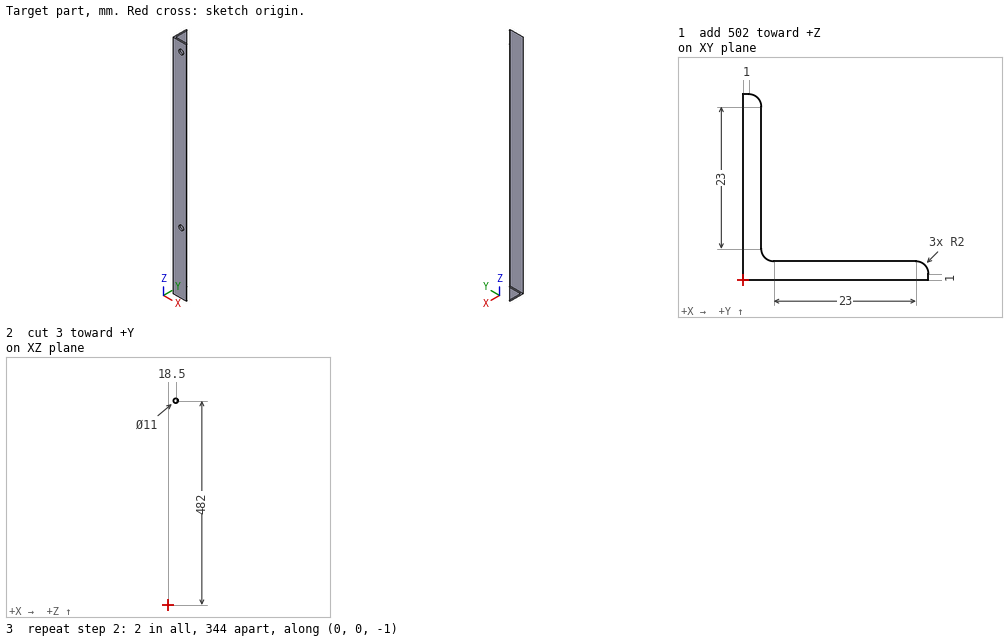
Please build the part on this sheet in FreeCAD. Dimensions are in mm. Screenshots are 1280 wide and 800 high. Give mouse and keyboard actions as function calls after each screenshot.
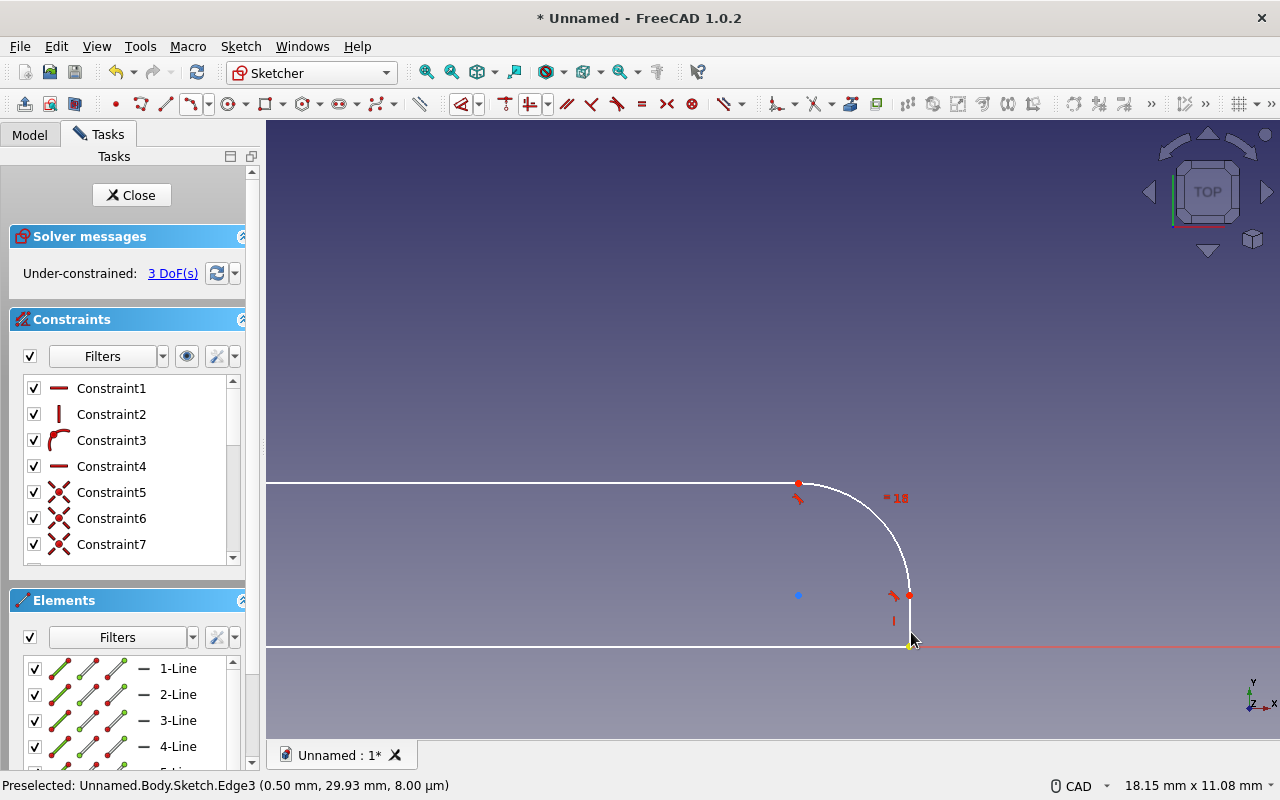
click(910, 631)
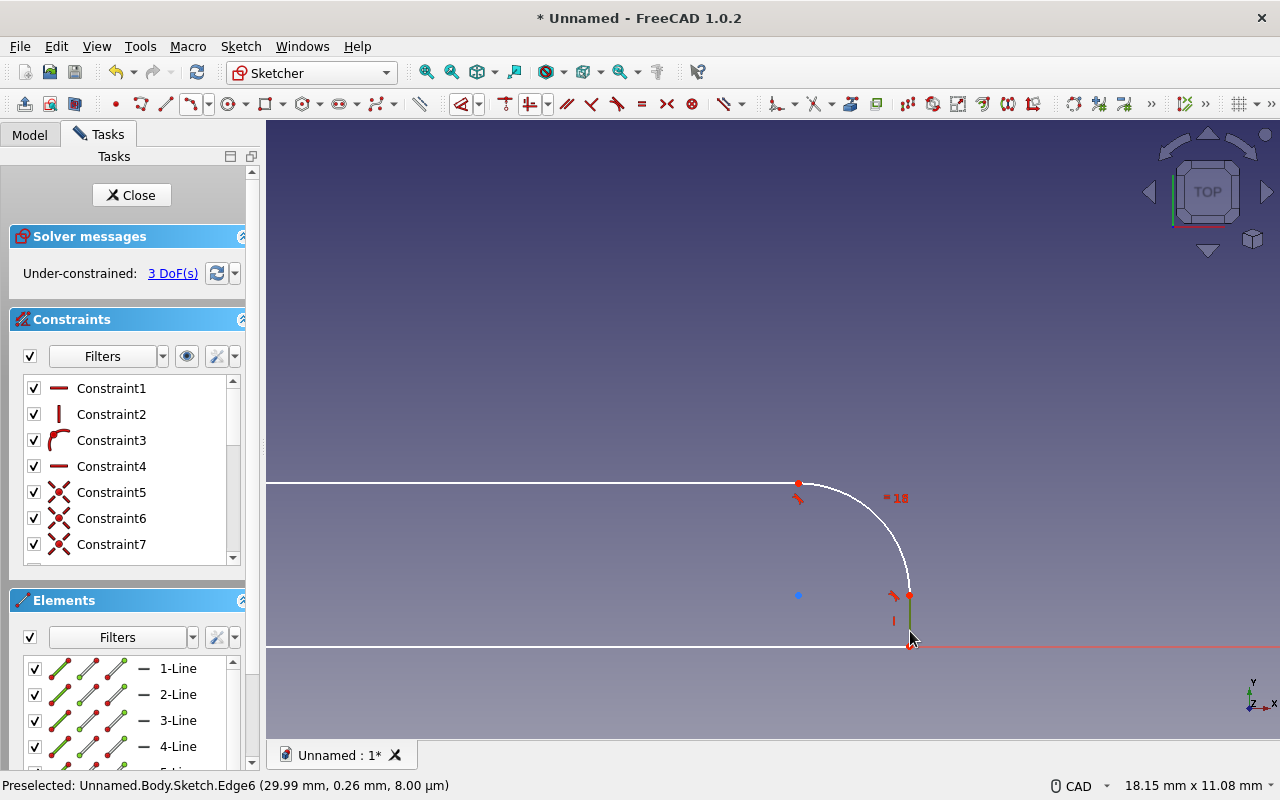
key(i)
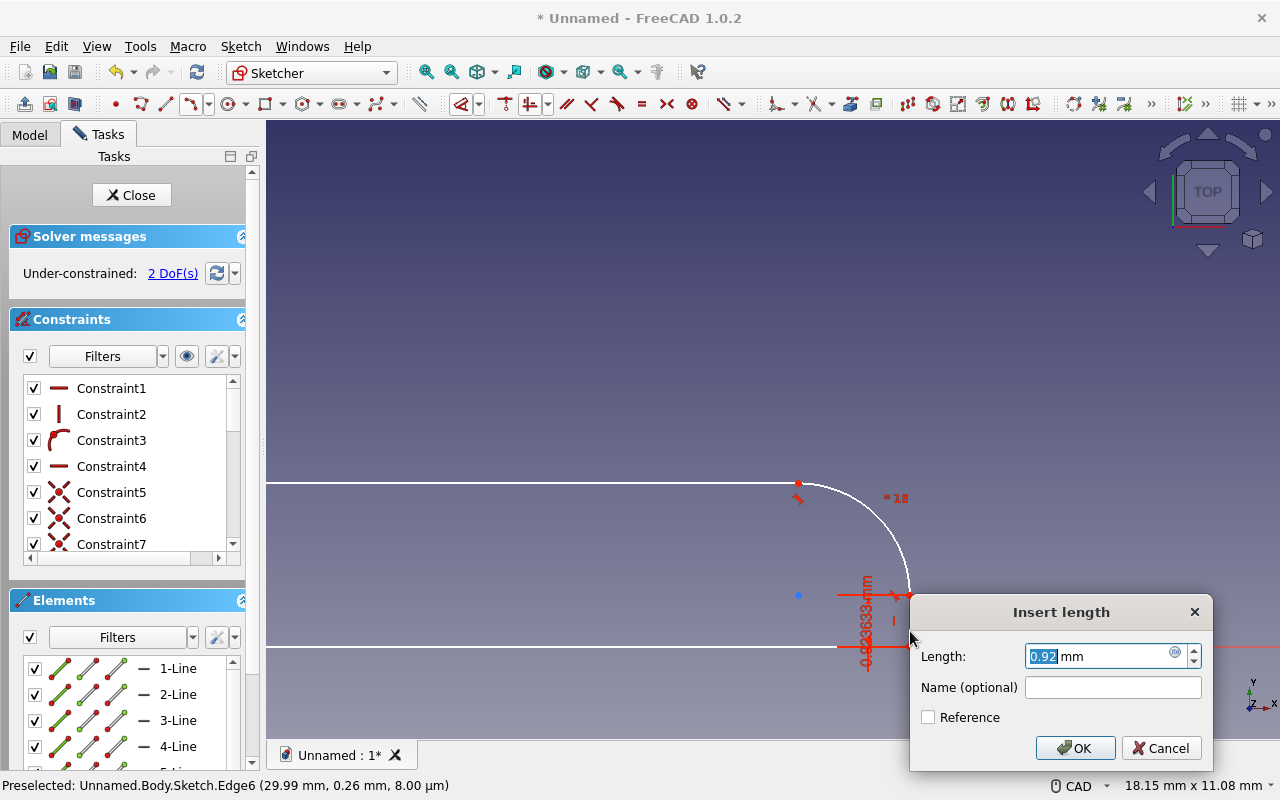
text(1)
key(Return)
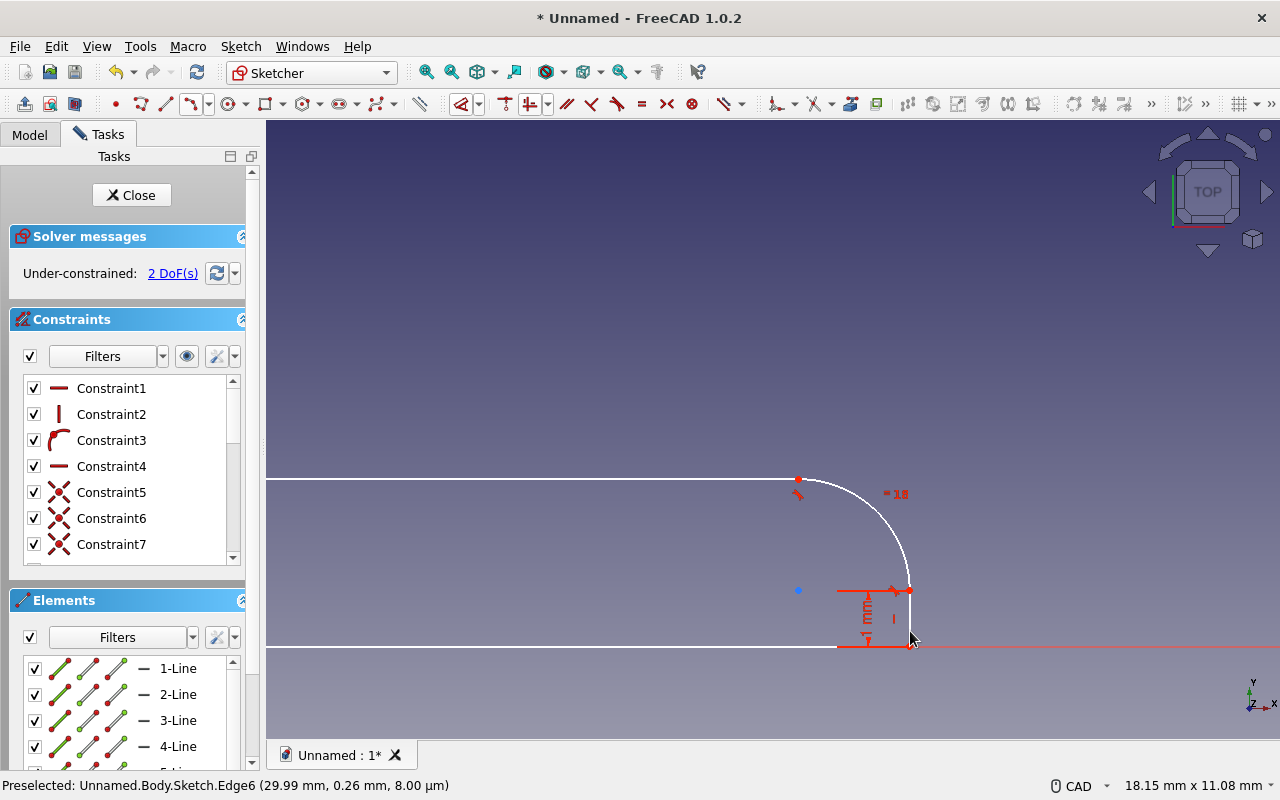
scroll(911, 633, down, 7)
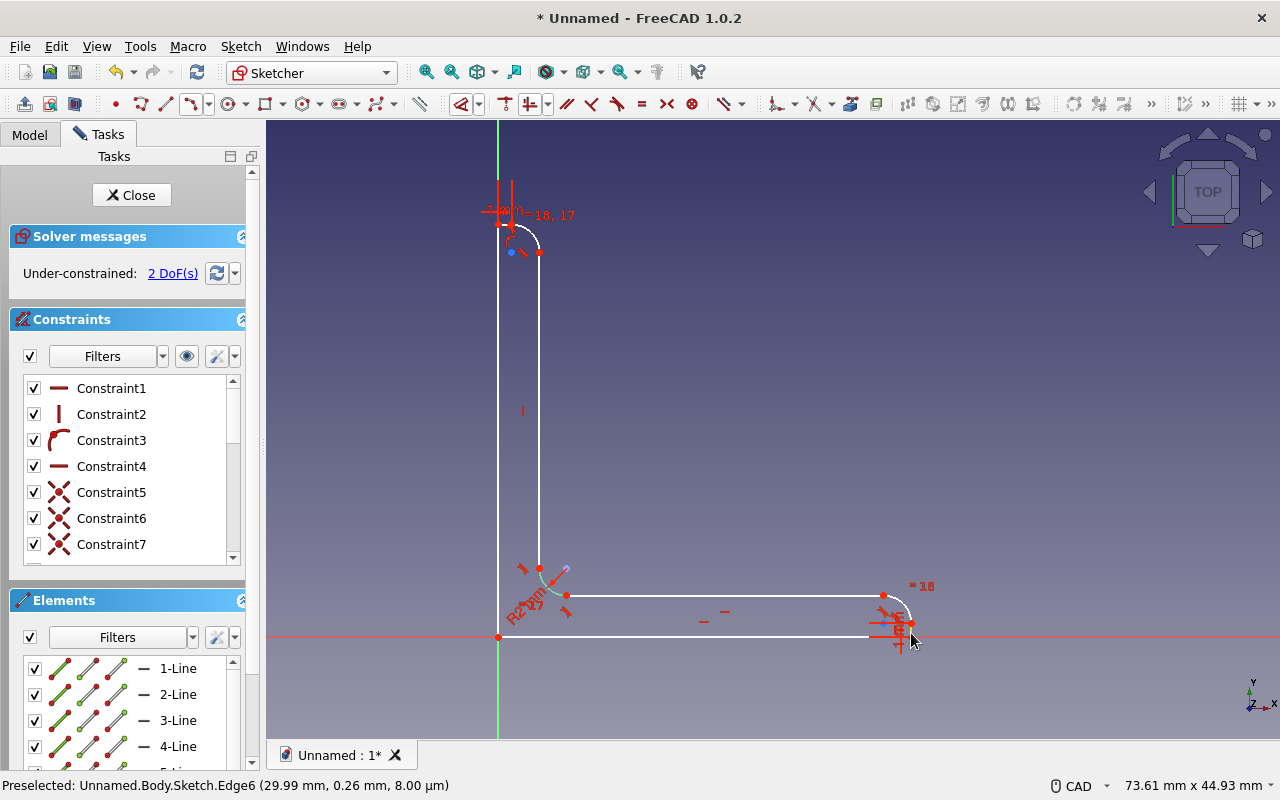
click(789, 596)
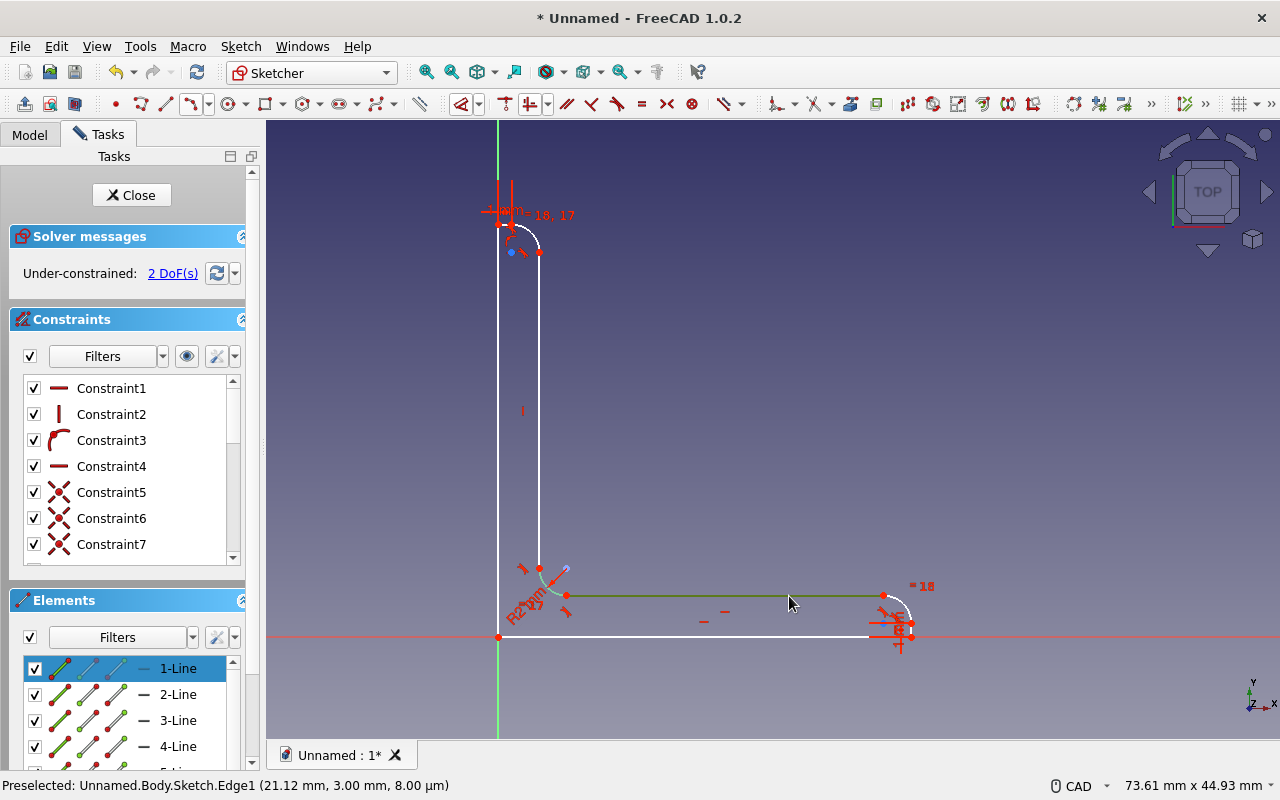
click(478, 104)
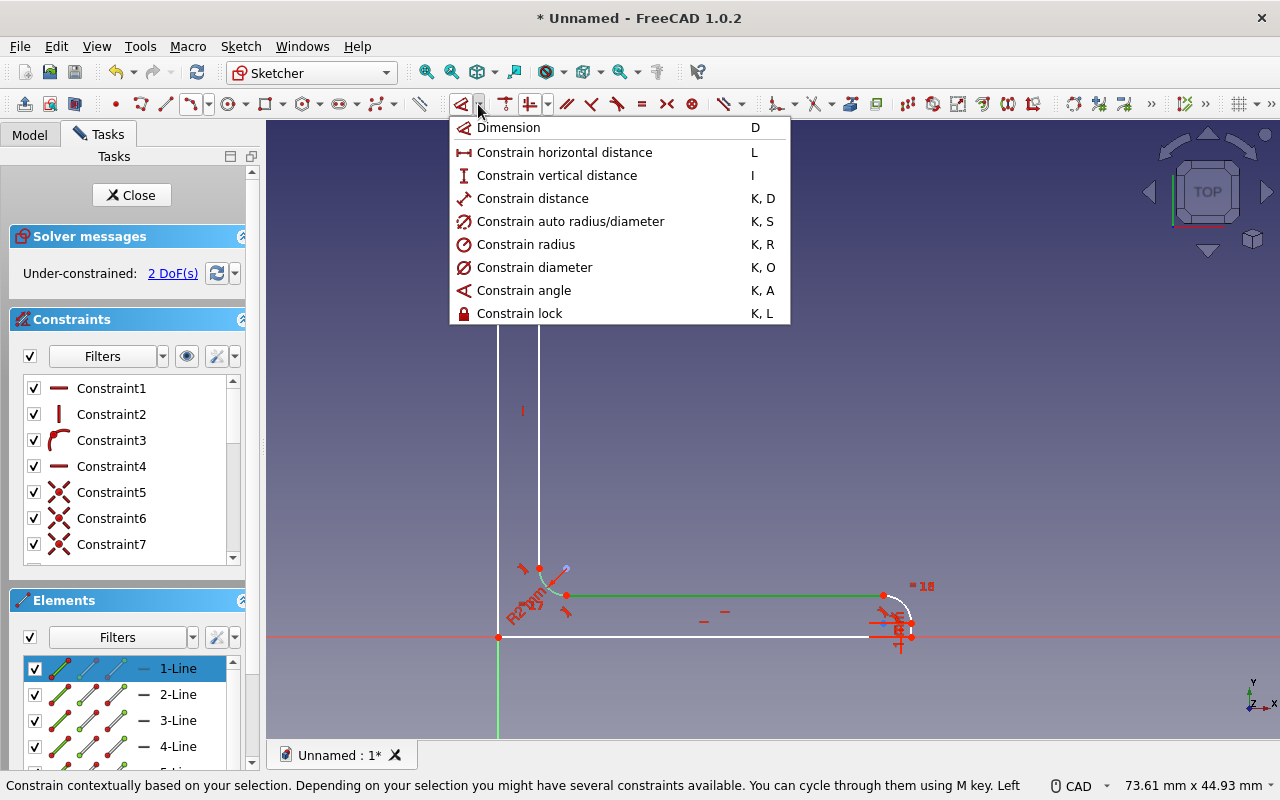
click(620, 152)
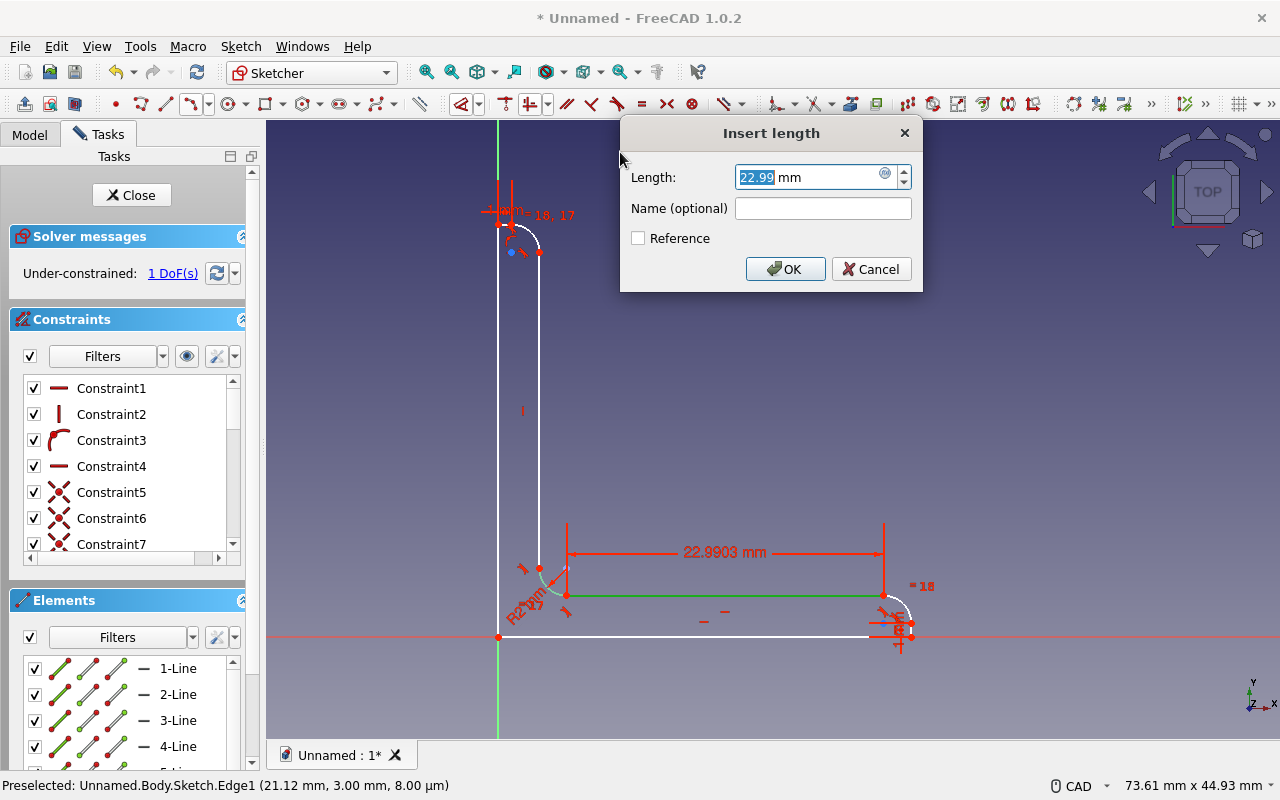
text(23)
key(Return)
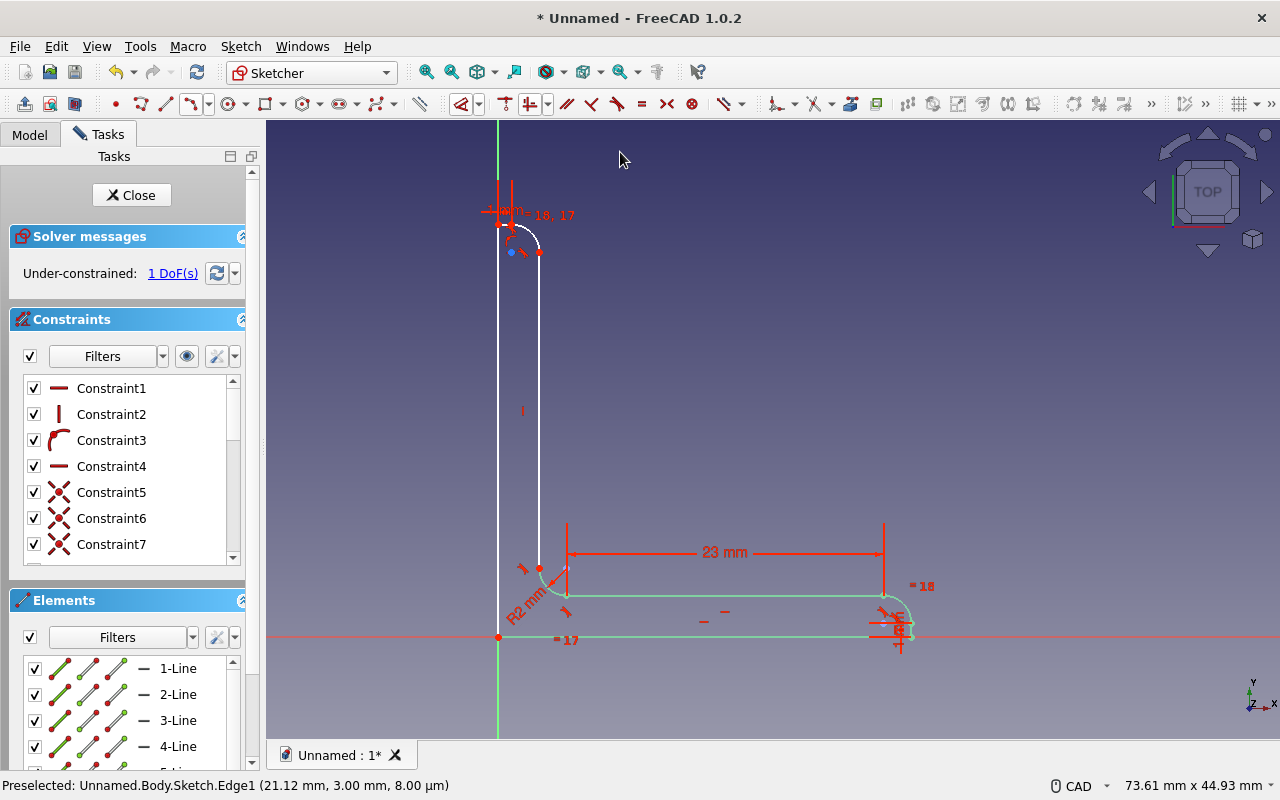
click(539, 473)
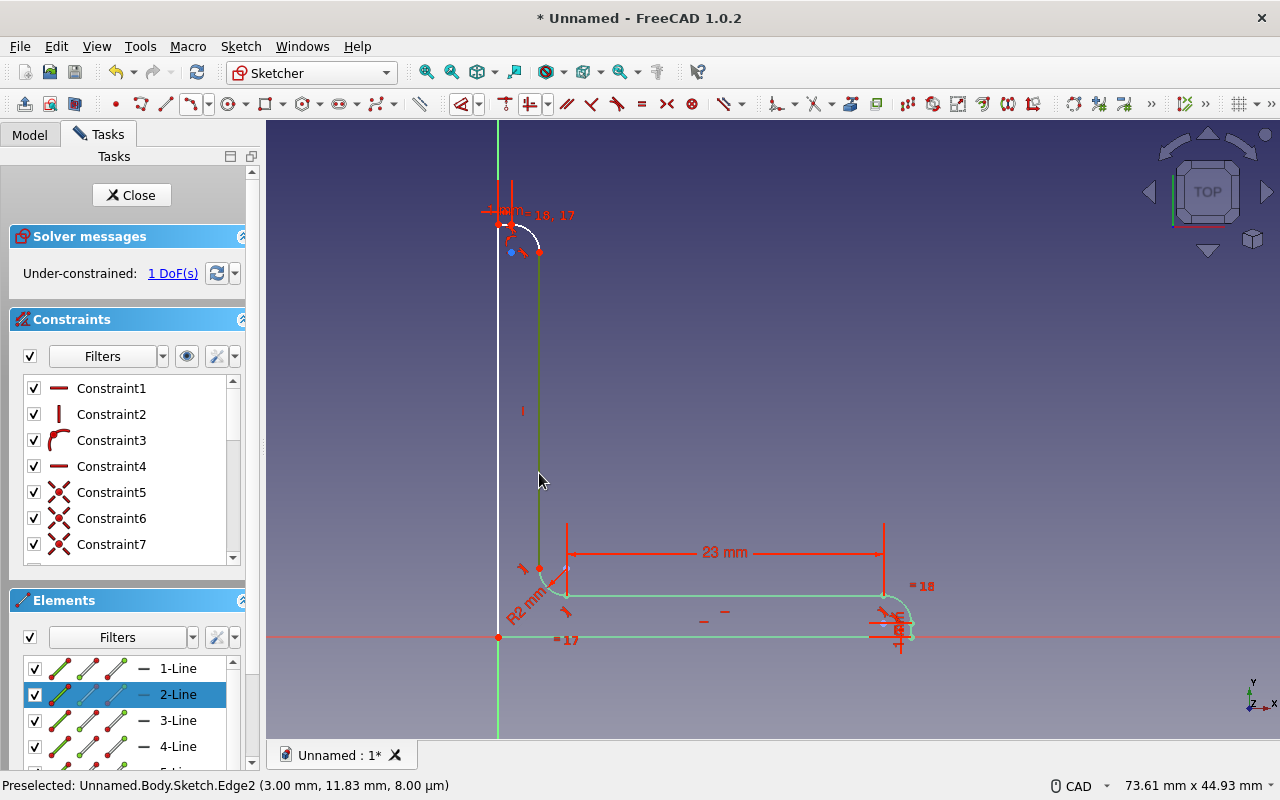
key(i)